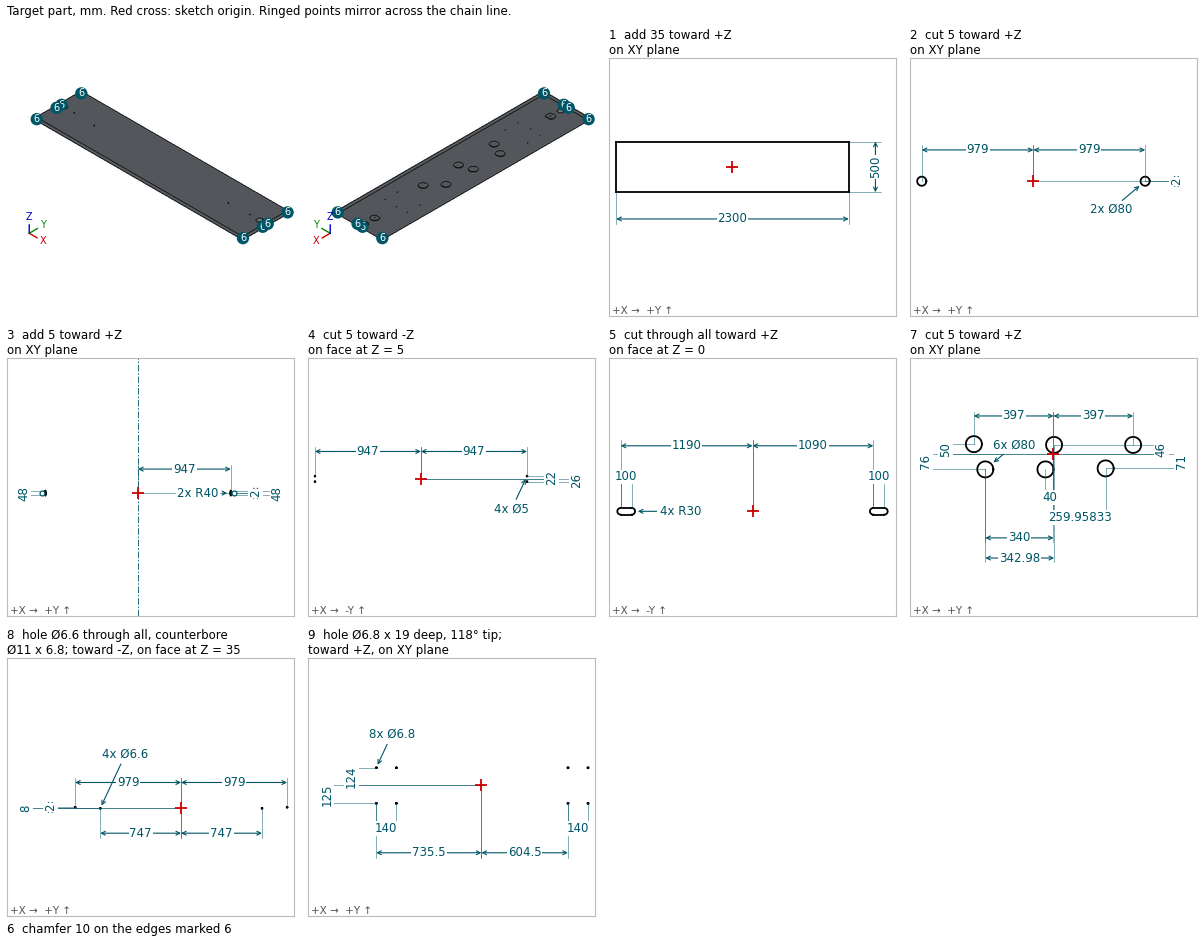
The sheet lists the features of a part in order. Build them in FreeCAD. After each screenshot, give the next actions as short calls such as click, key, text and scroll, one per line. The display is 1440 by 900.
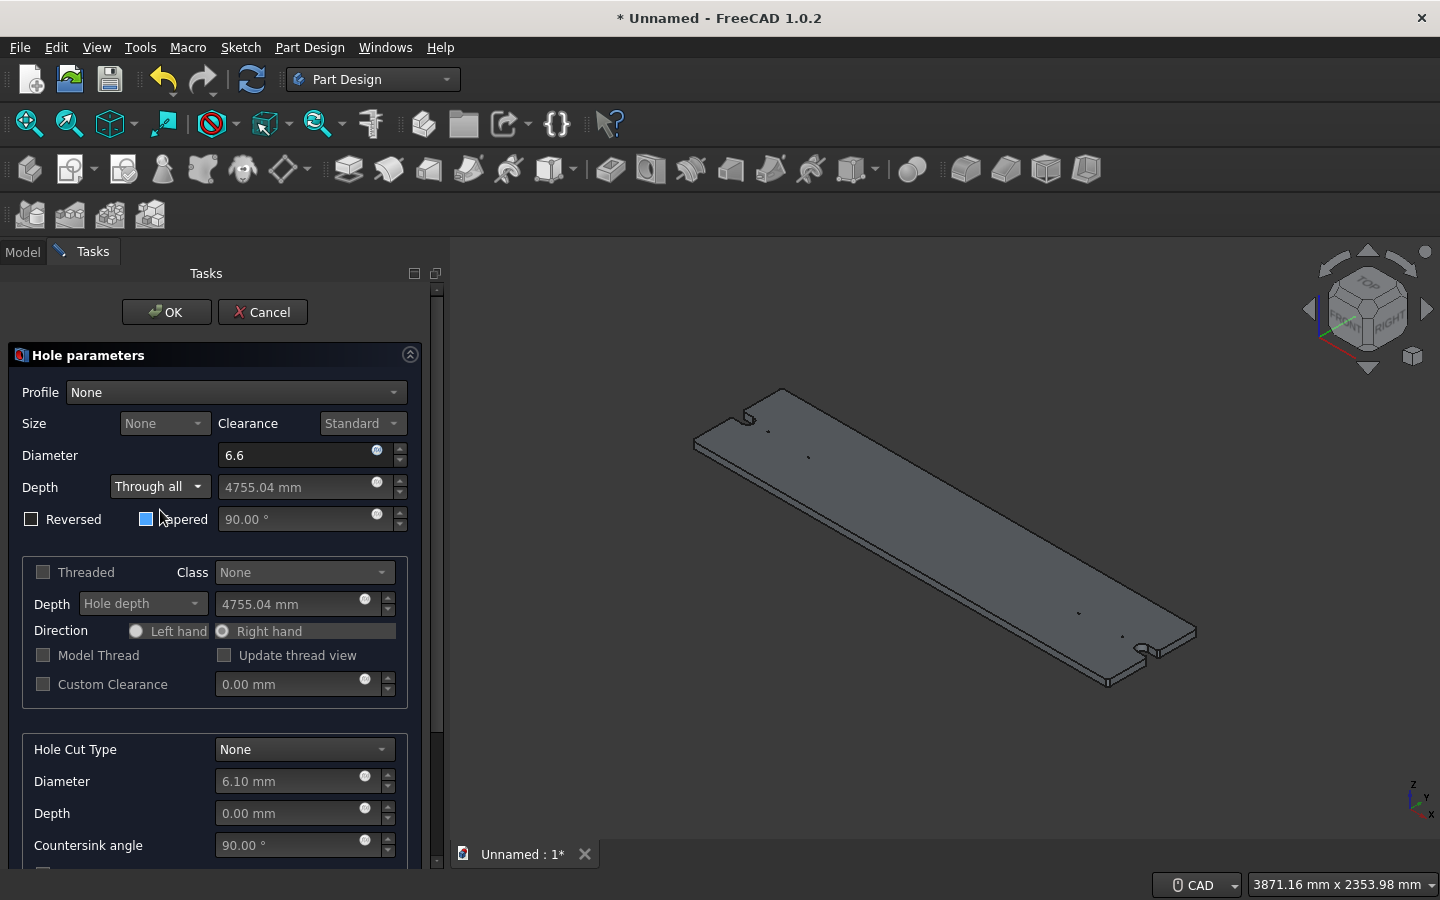
click(306, 750)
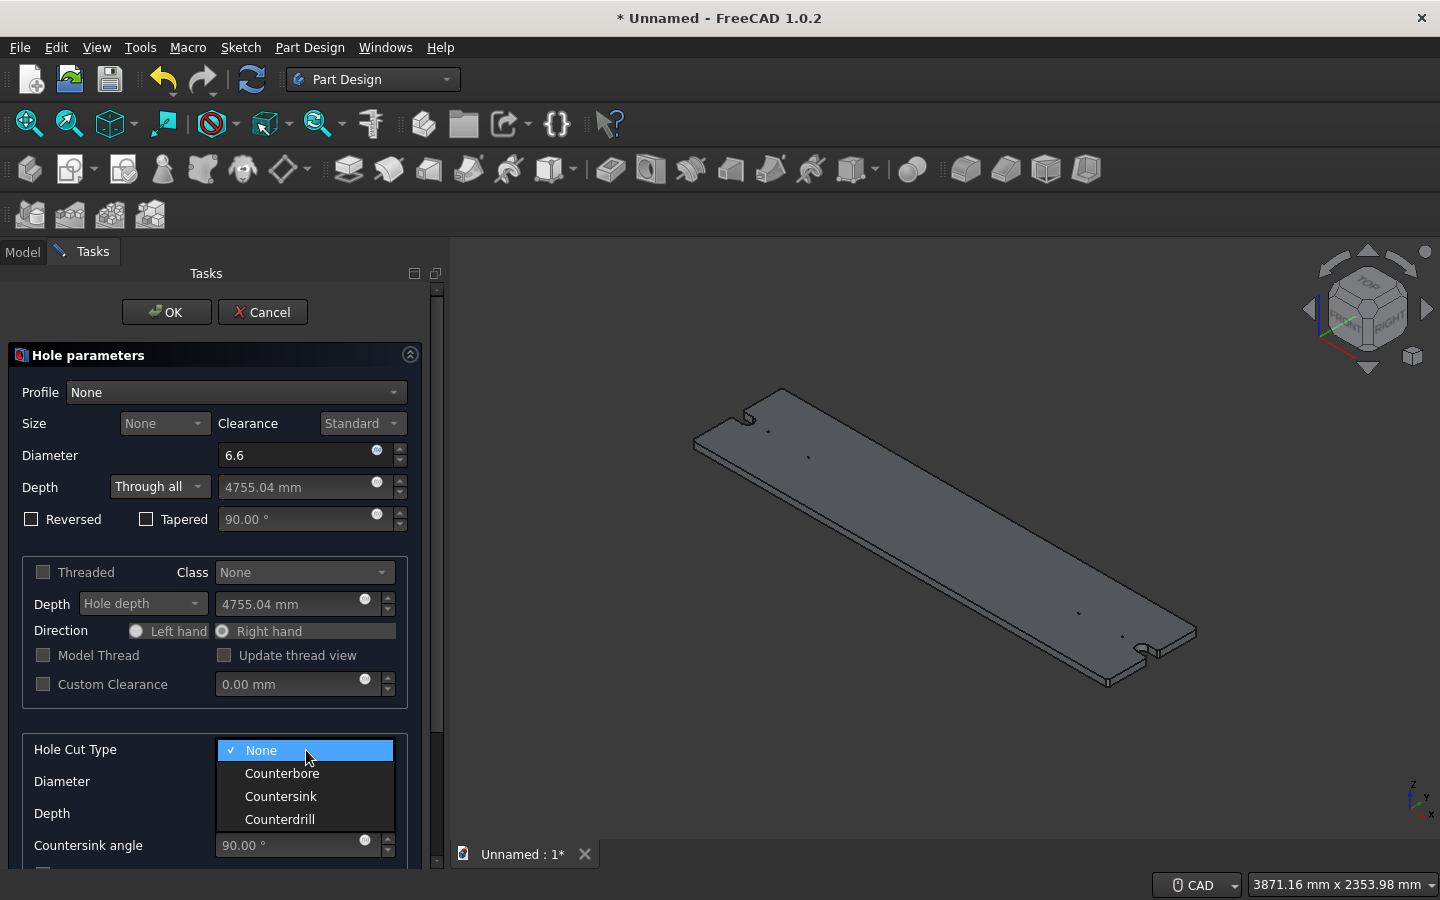
click(304, 774)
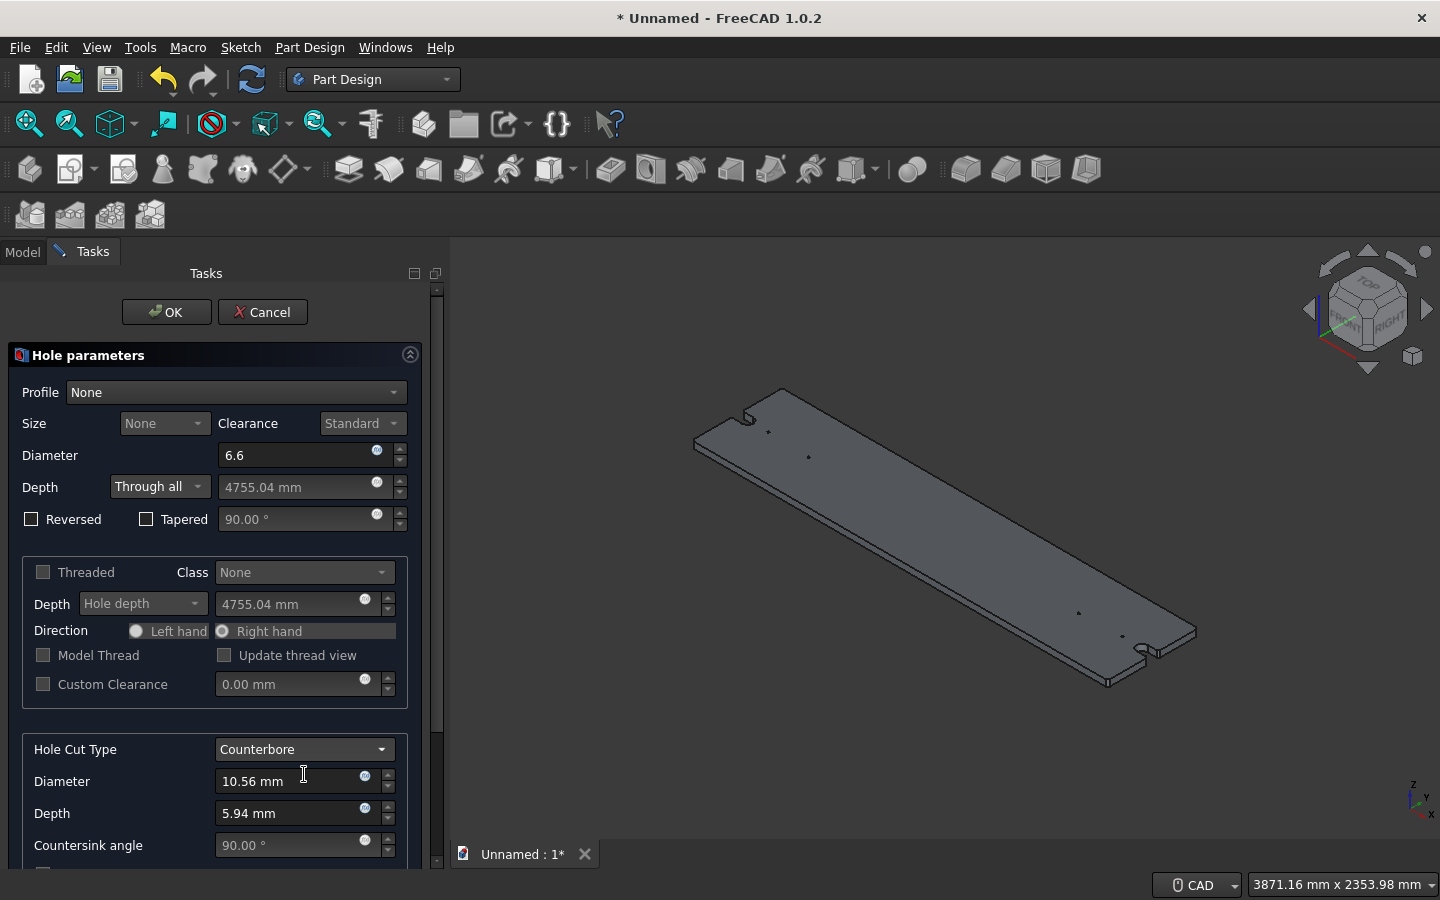
triple_click(298, 781)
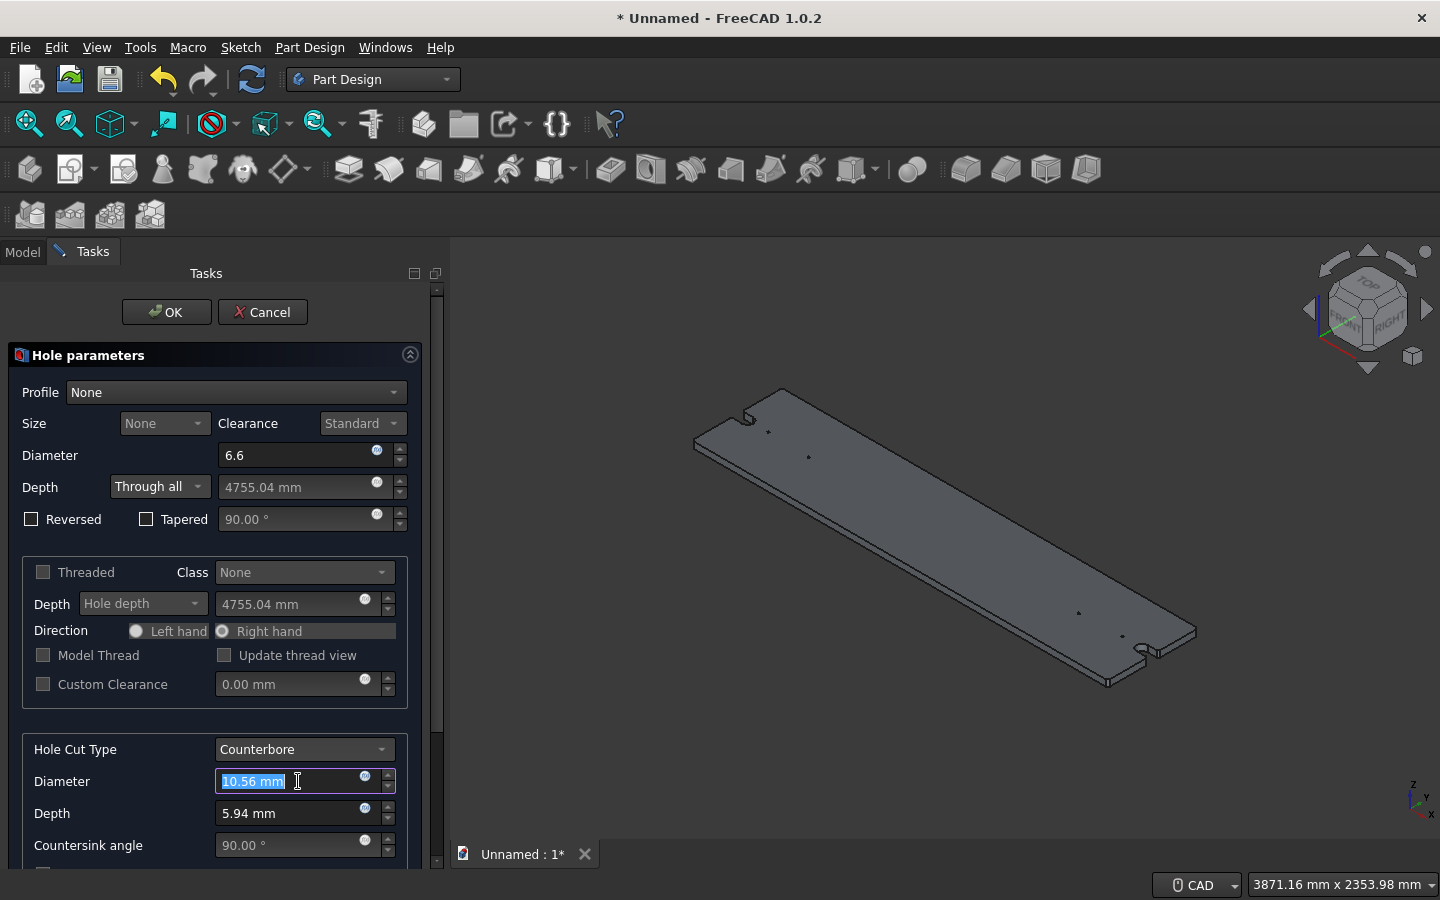
text(11)
key(Tab)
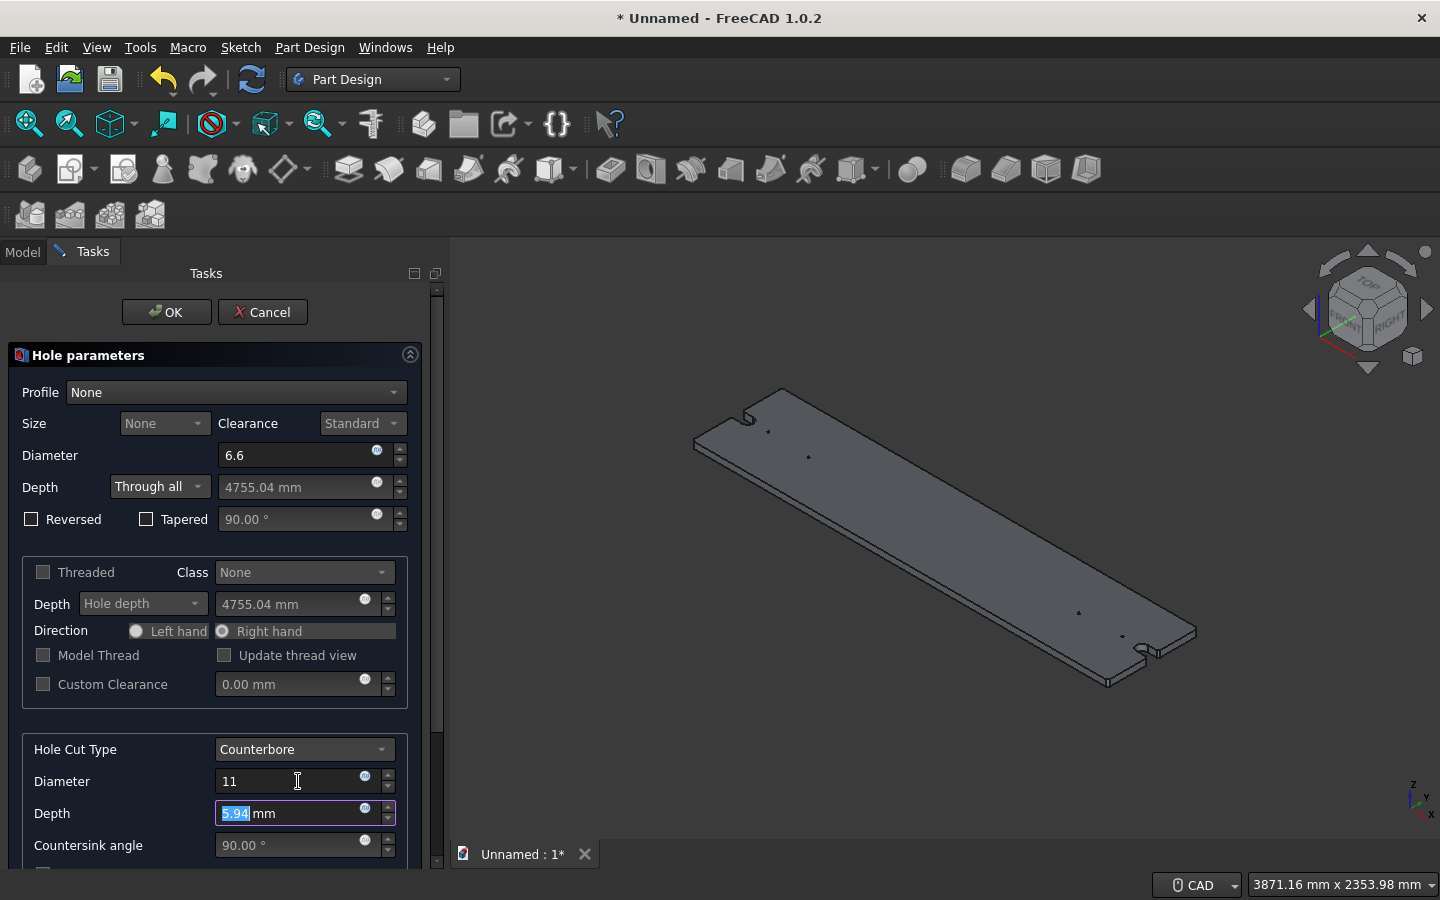
text(6.8)
key(Tab)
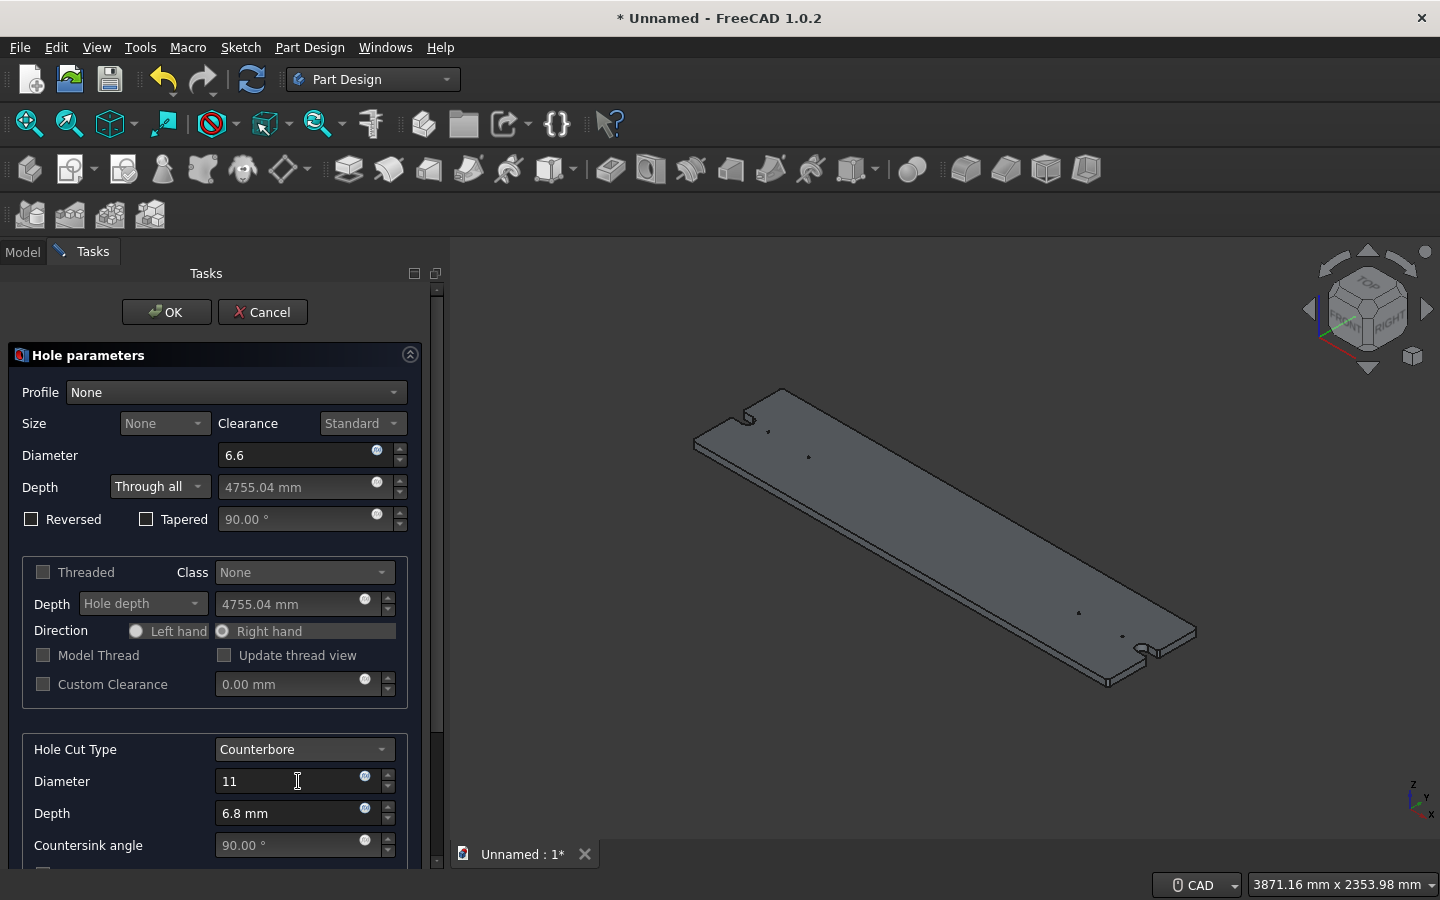
click(167, 312)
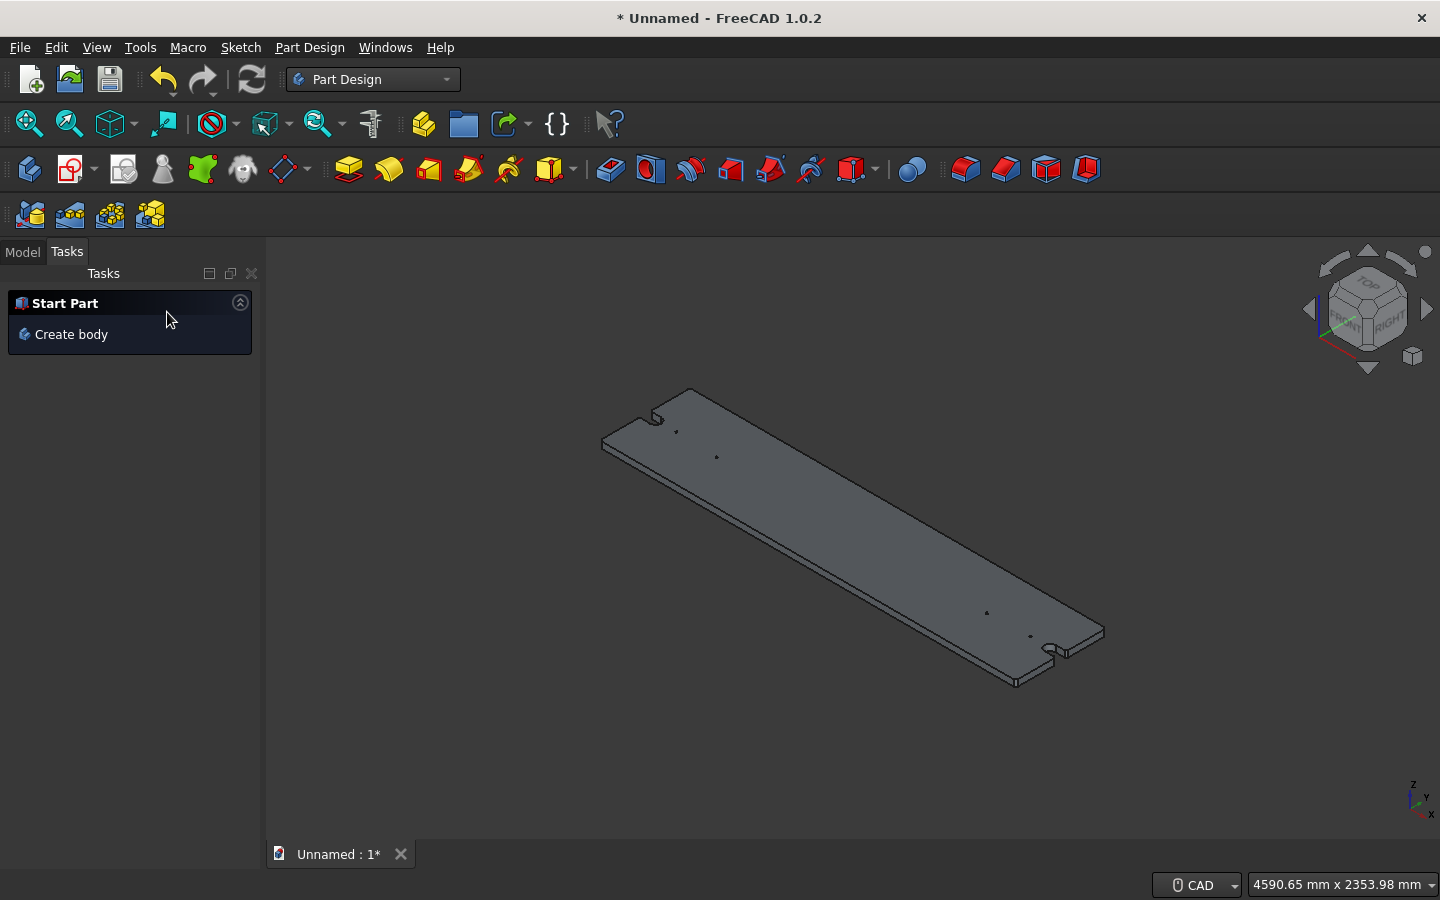
click(70, 170)